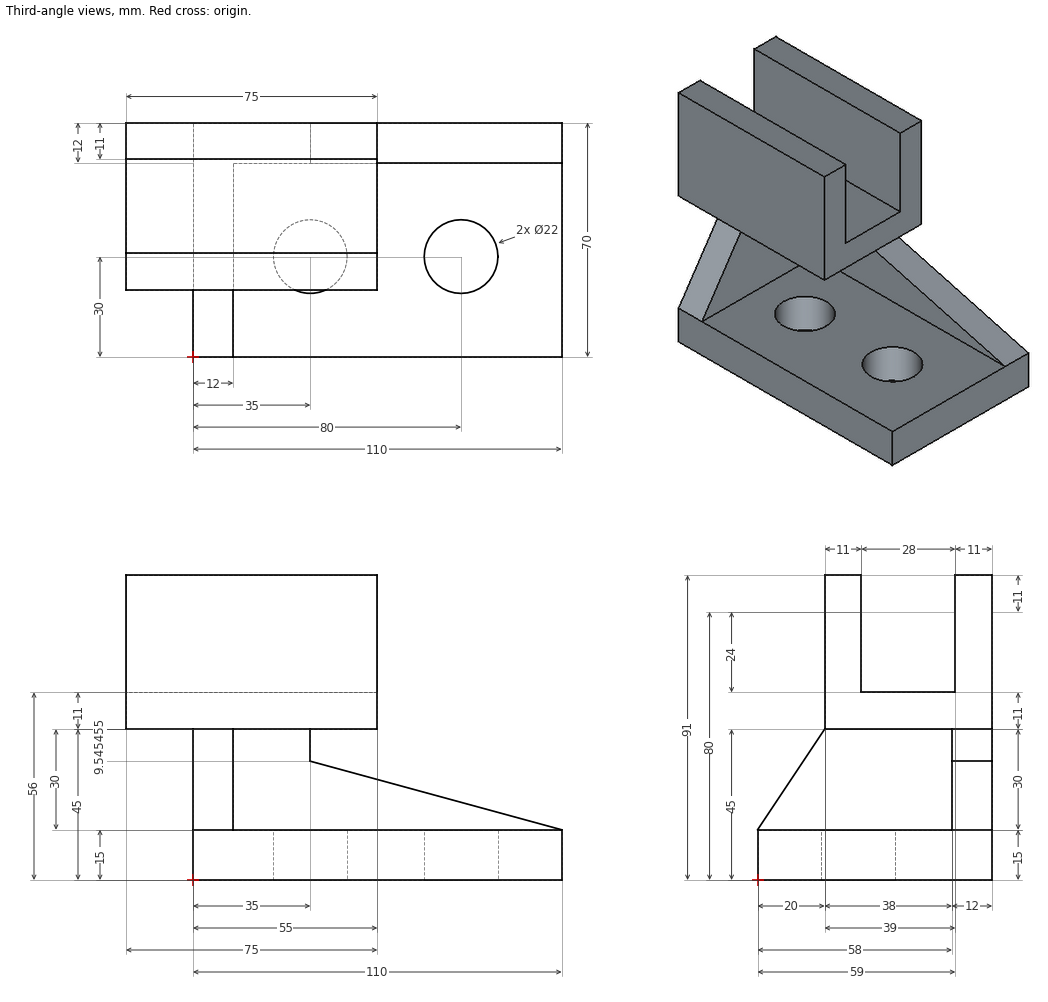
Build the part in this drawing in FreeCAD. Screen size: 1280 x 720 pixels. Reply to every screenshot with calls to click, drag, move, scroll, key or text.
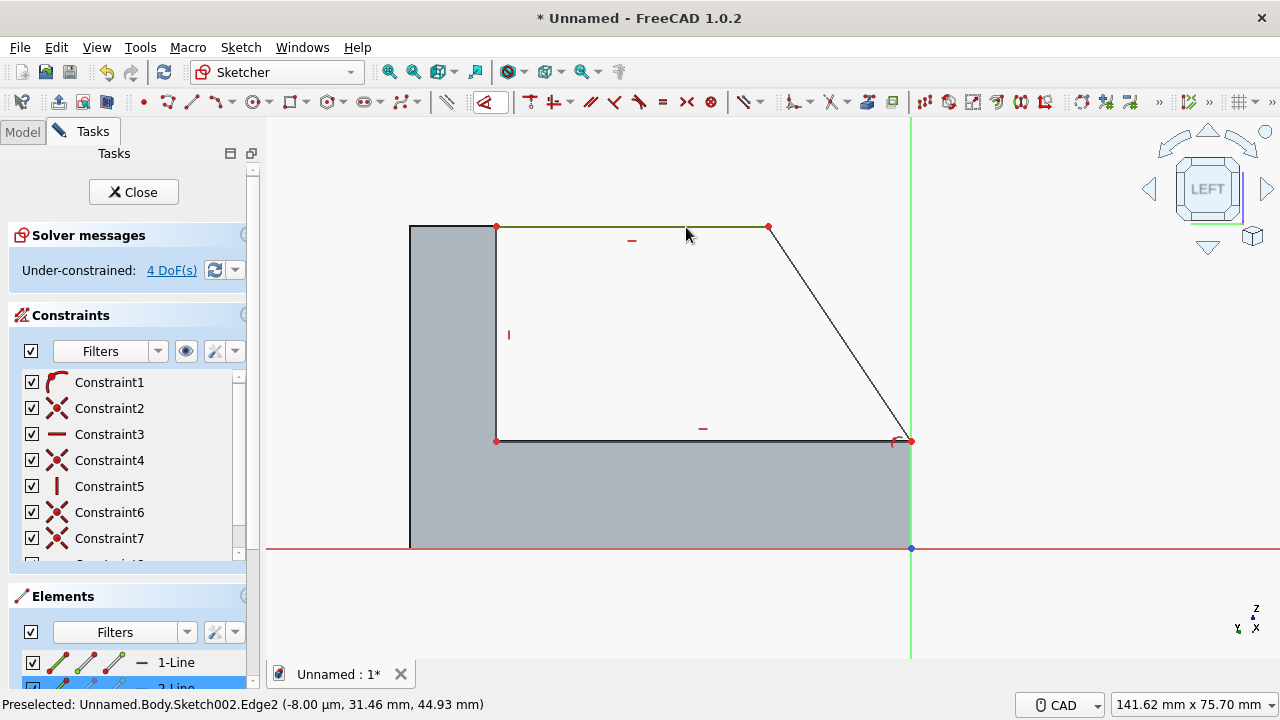
key(l)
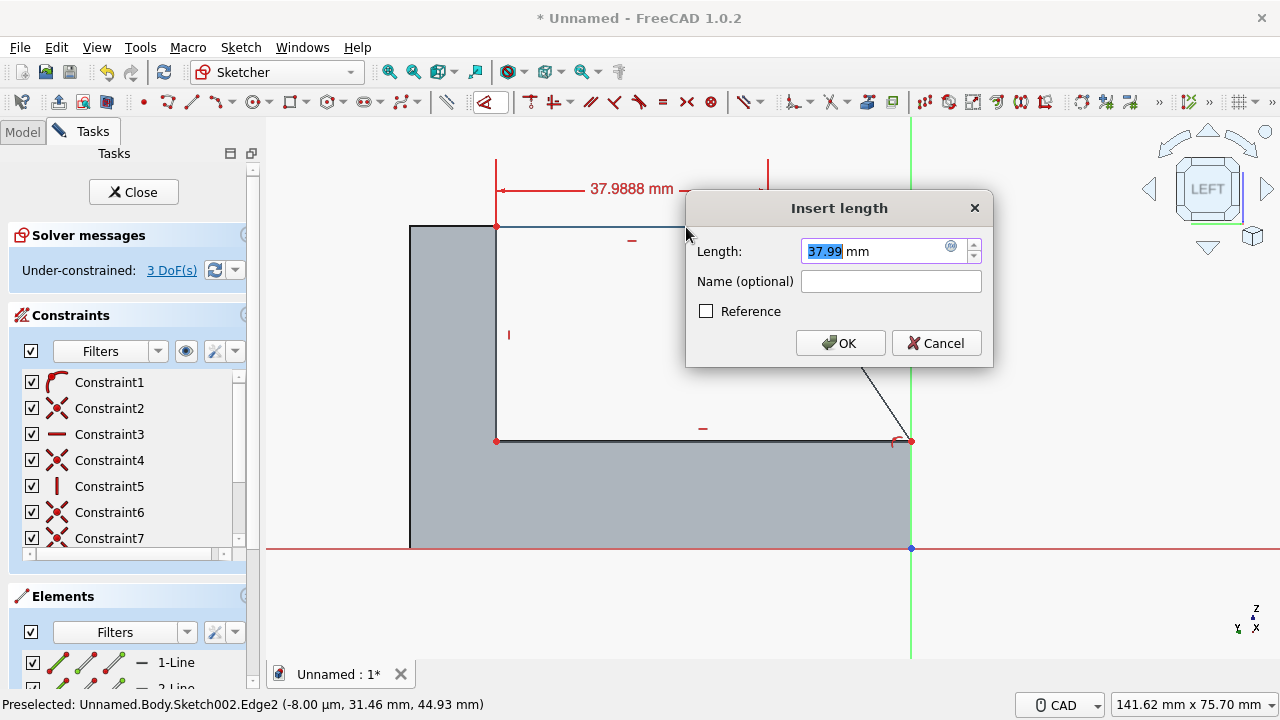
text(38)
key(Return)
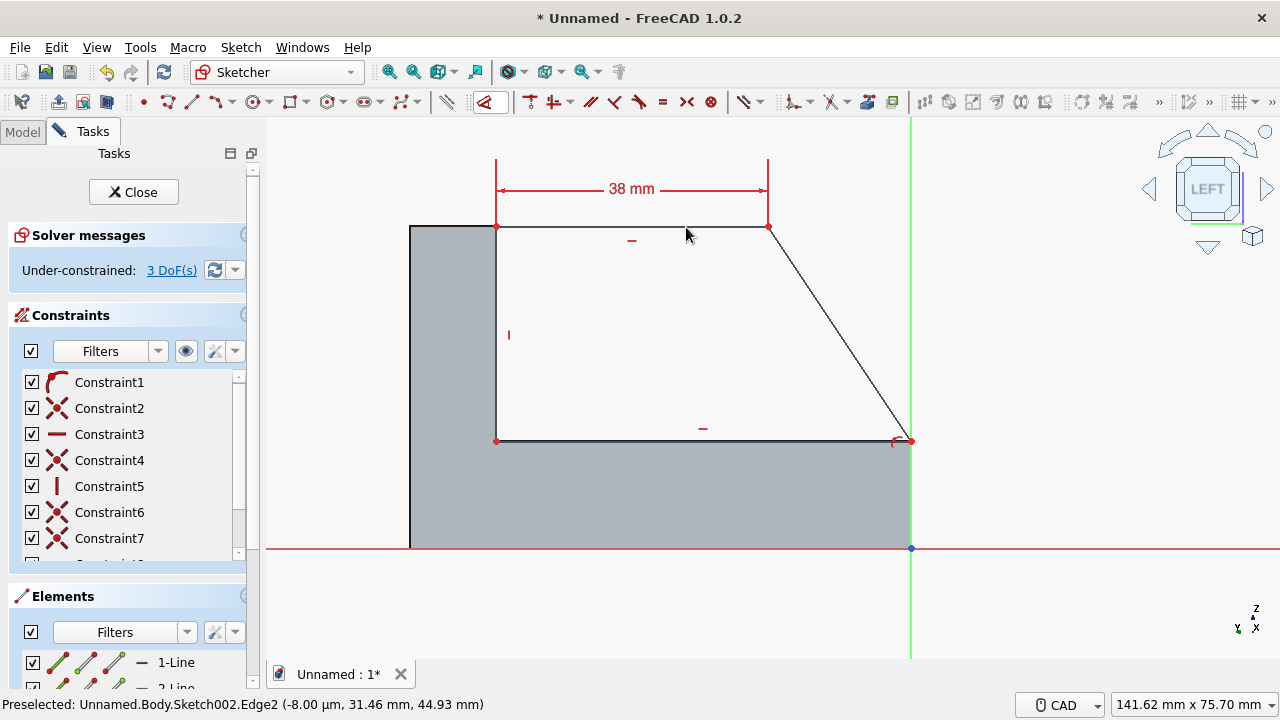
click(496, 291)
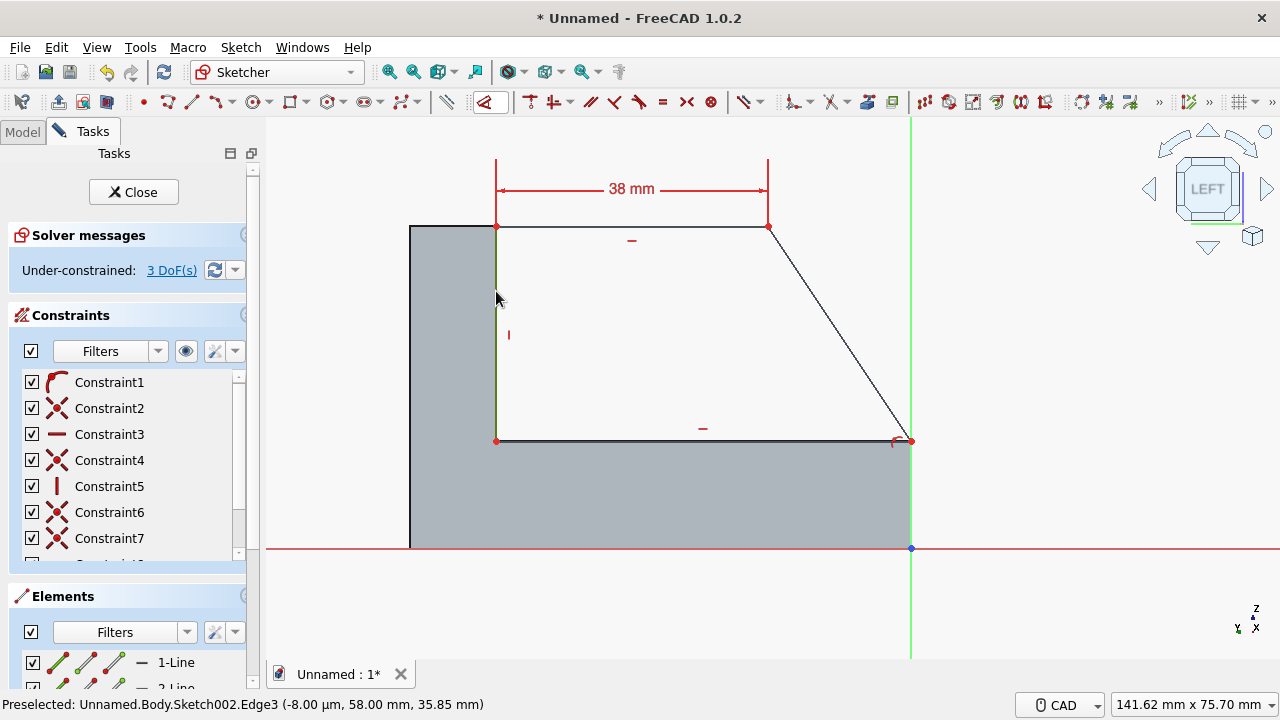
click(502, 102)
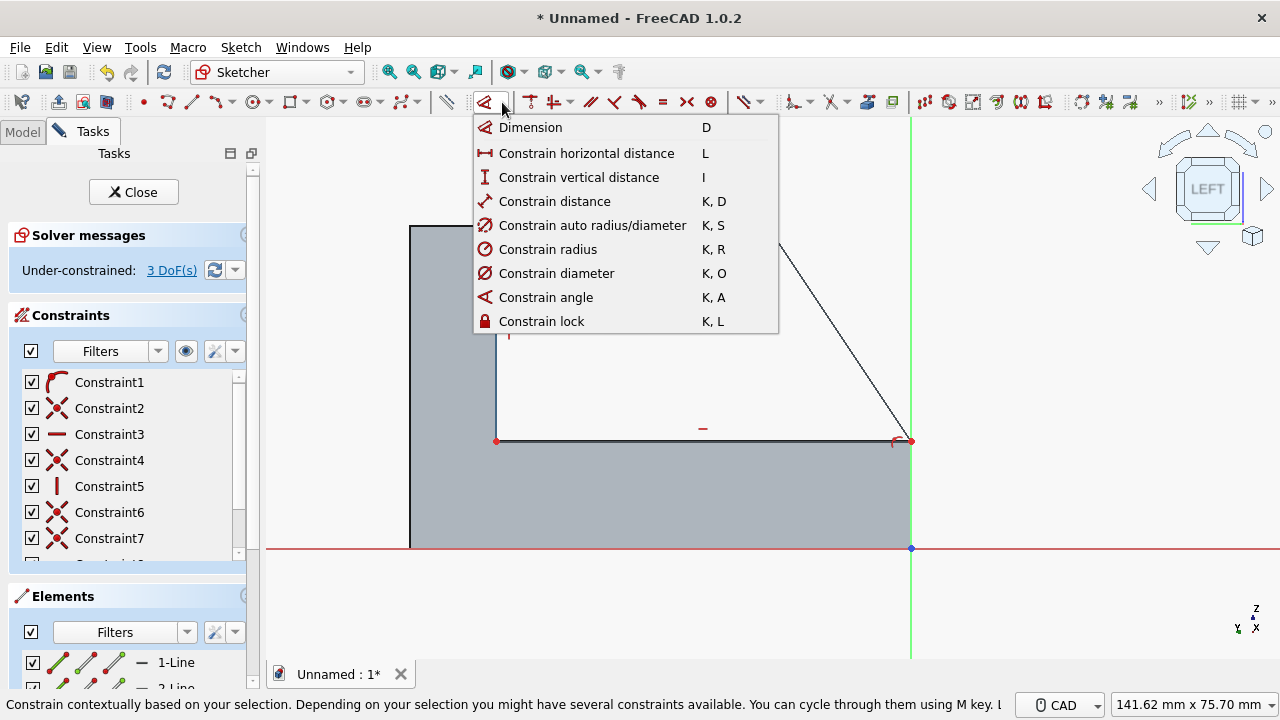
click(626, 177)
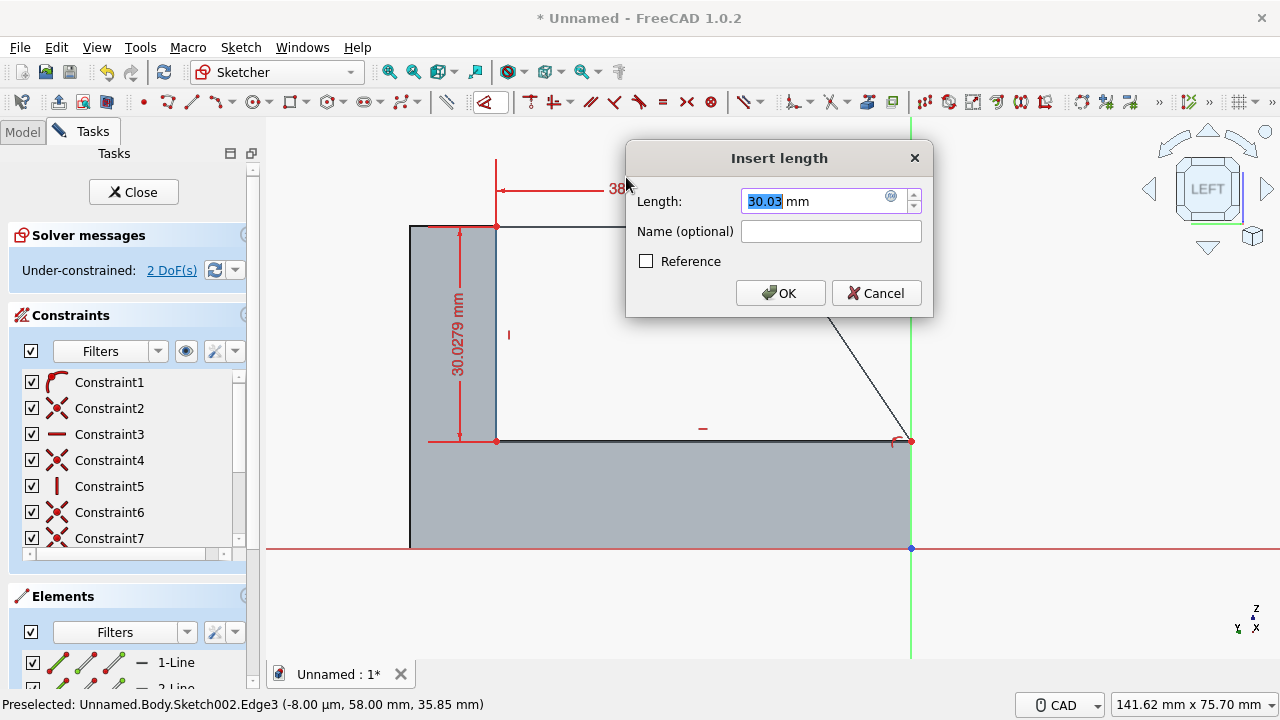
text(30)
key(Return)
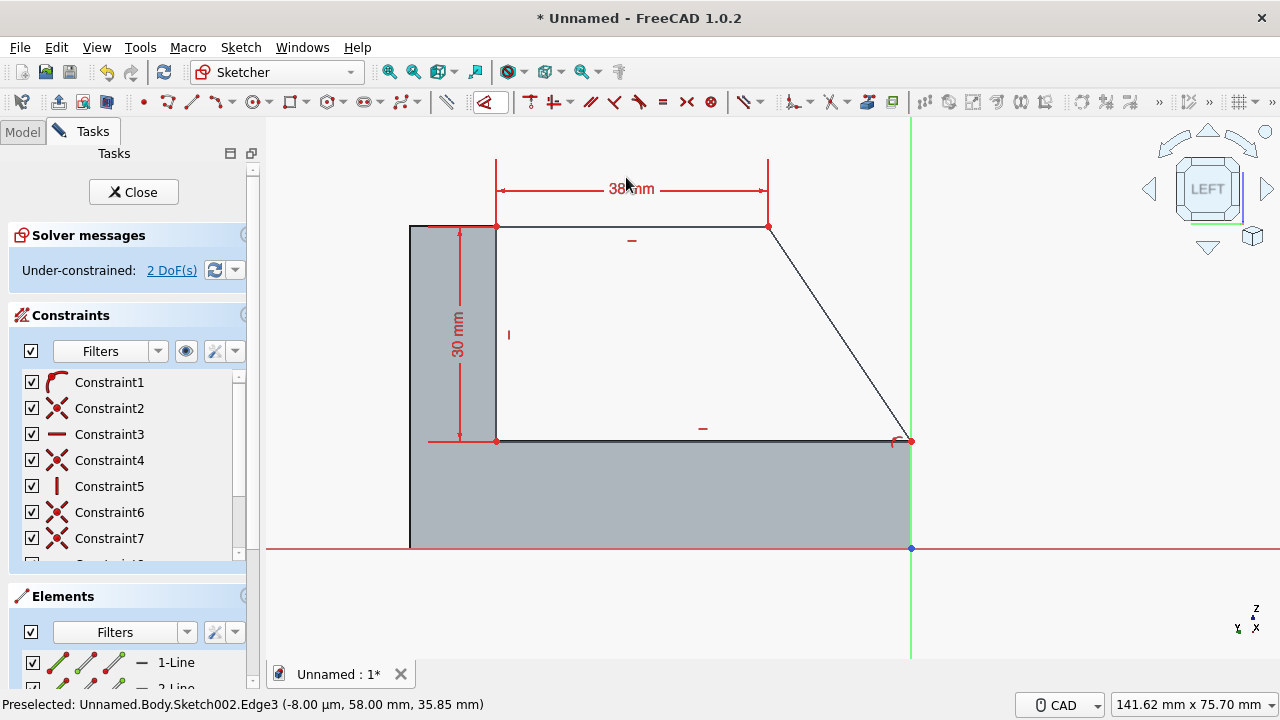
click(621, 442)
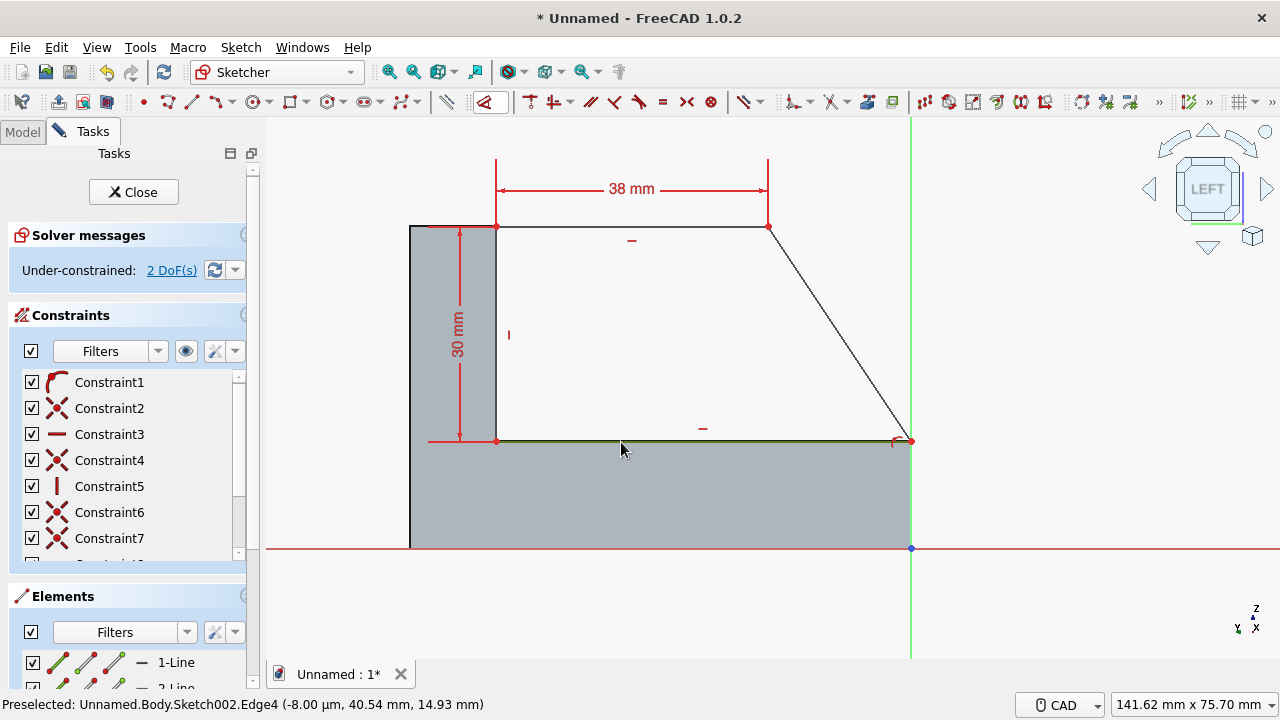
key(l)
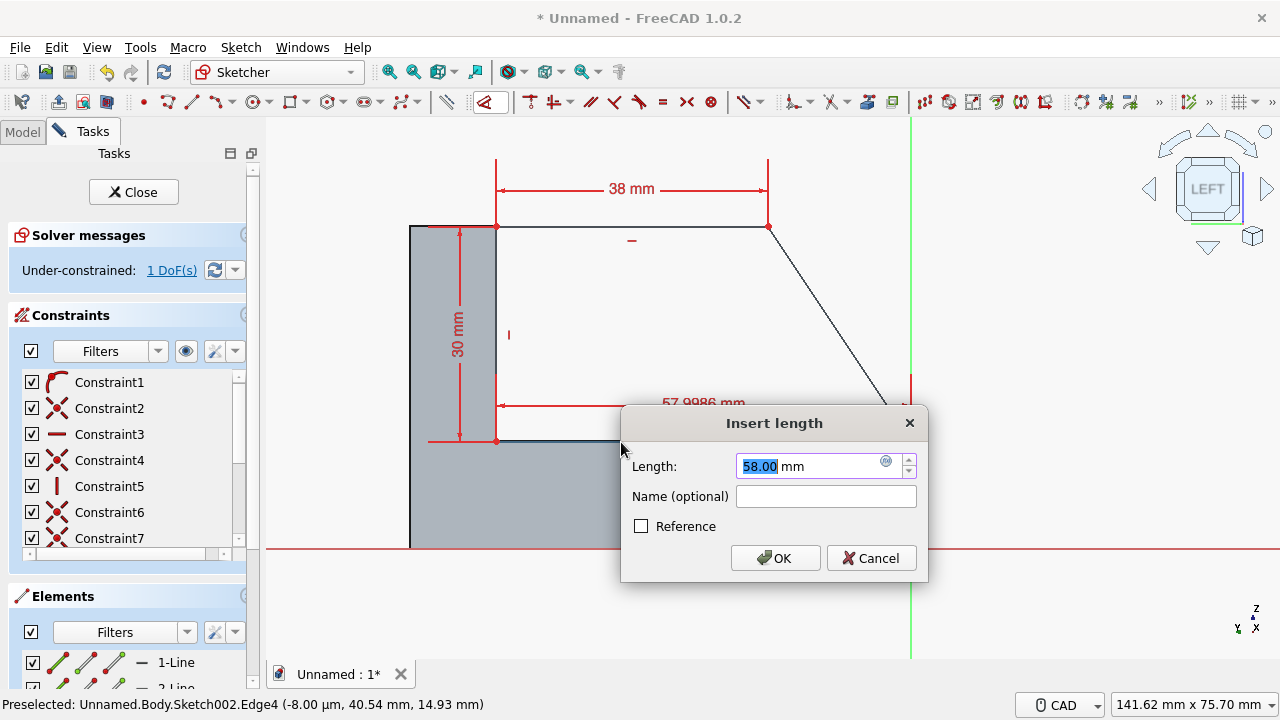
text(58)
key(Return)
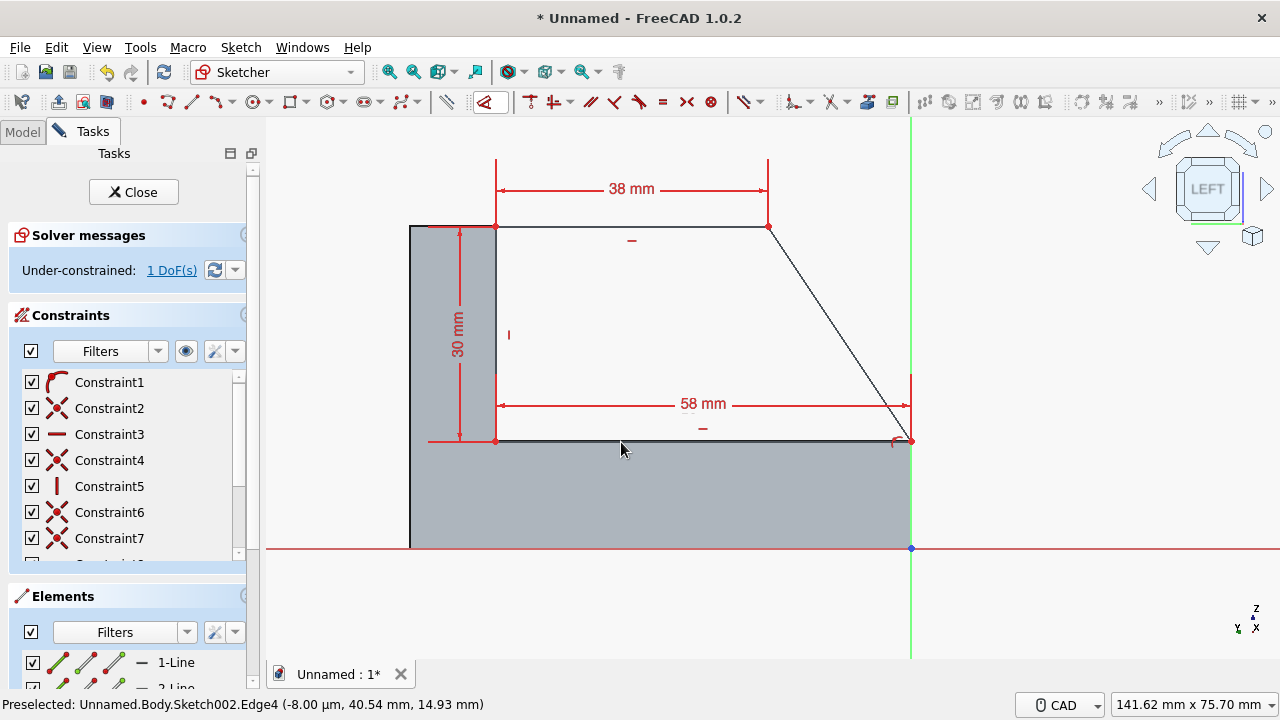
click(911, 442)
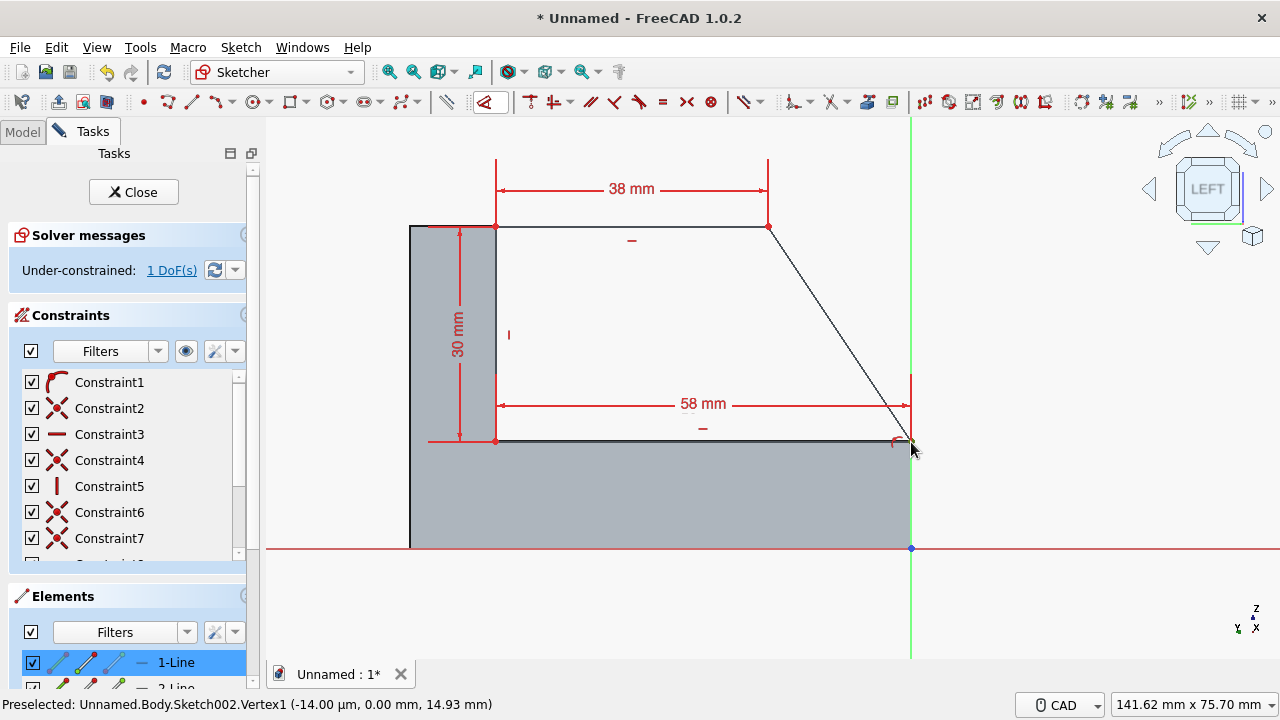
key(i)